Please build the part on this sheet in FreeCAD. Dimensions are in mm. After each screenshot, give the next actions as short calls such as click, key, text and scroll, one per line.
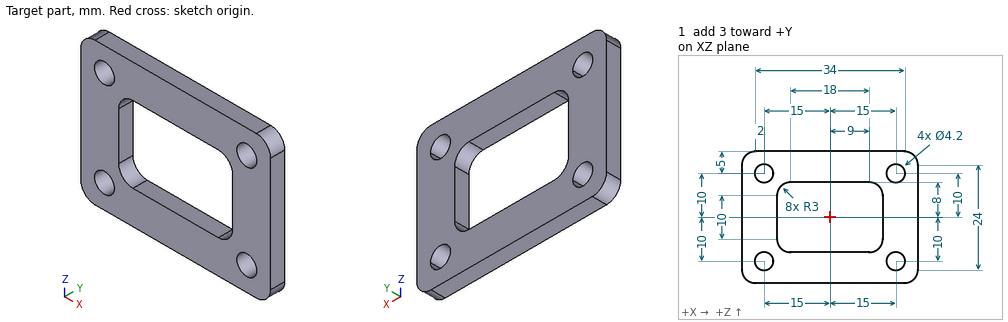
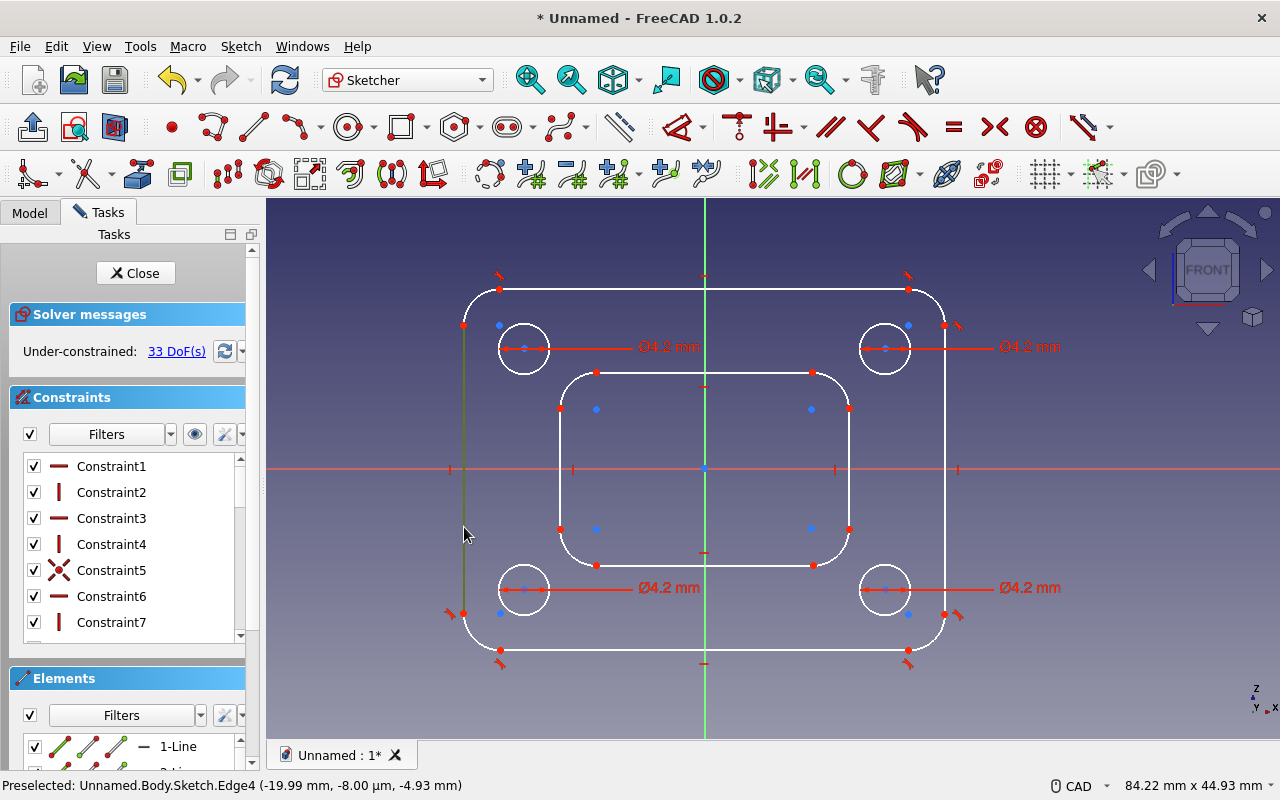
click(484, 293)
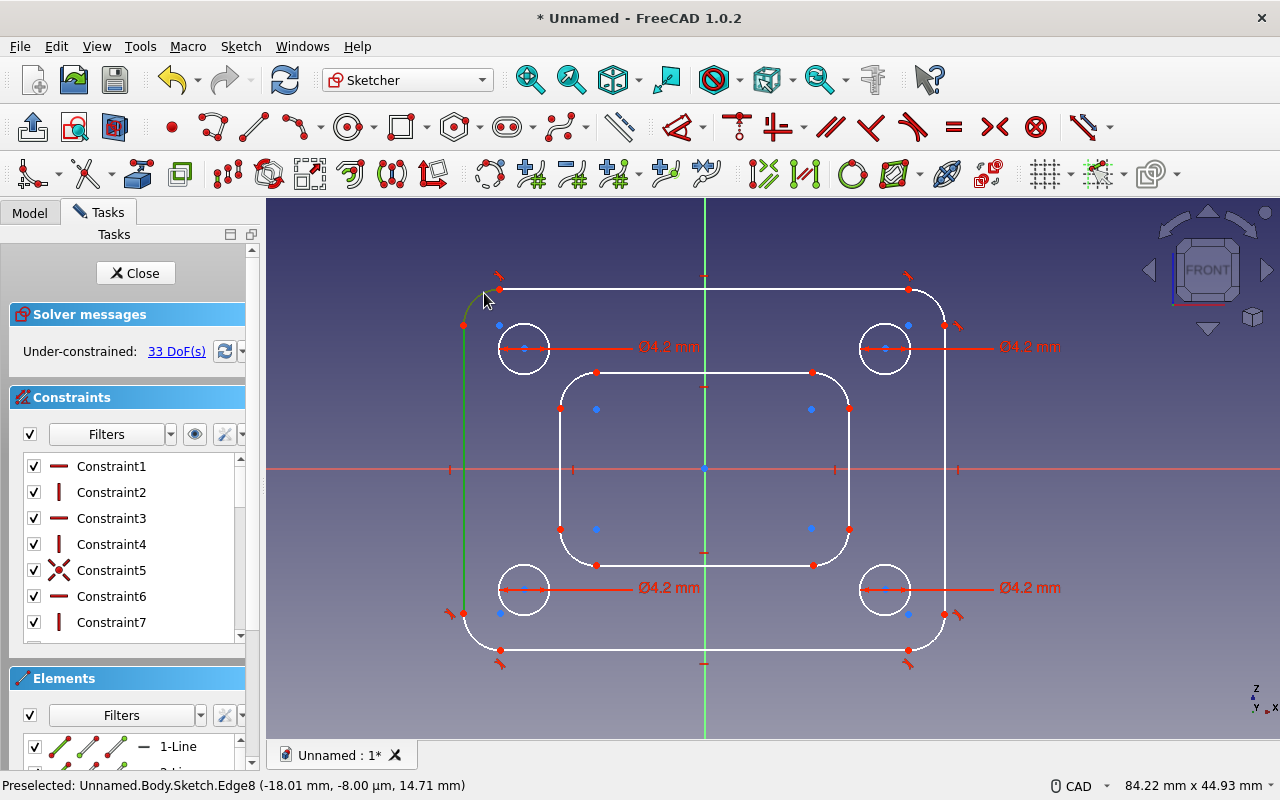
key(t)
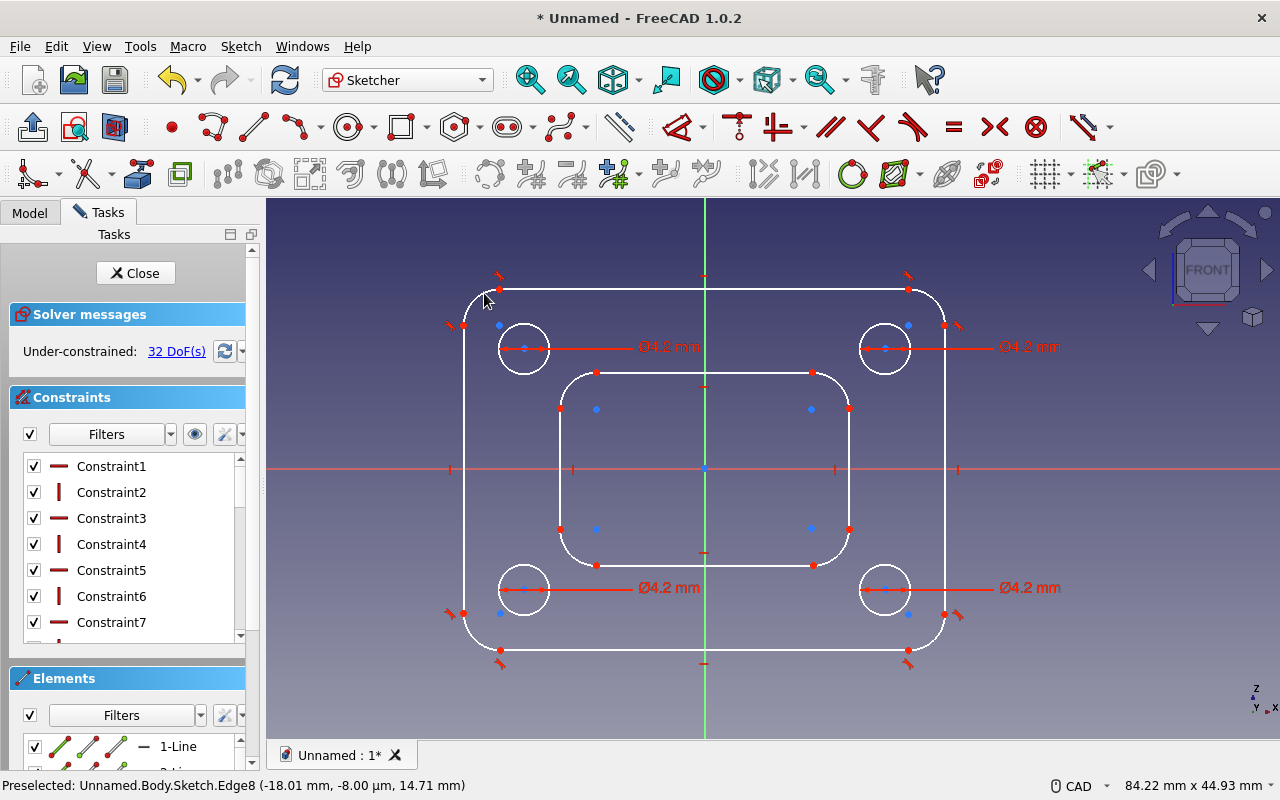
click(748, 373)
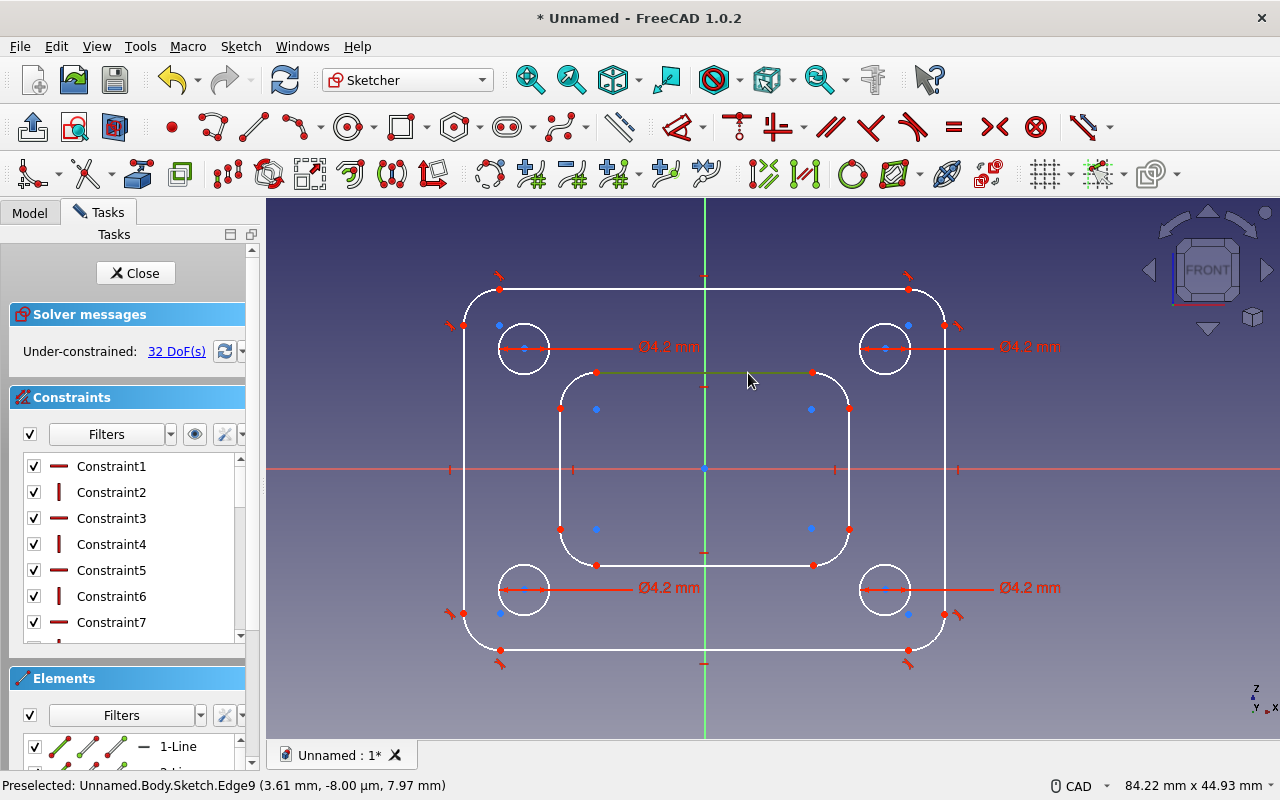
click(580, 377)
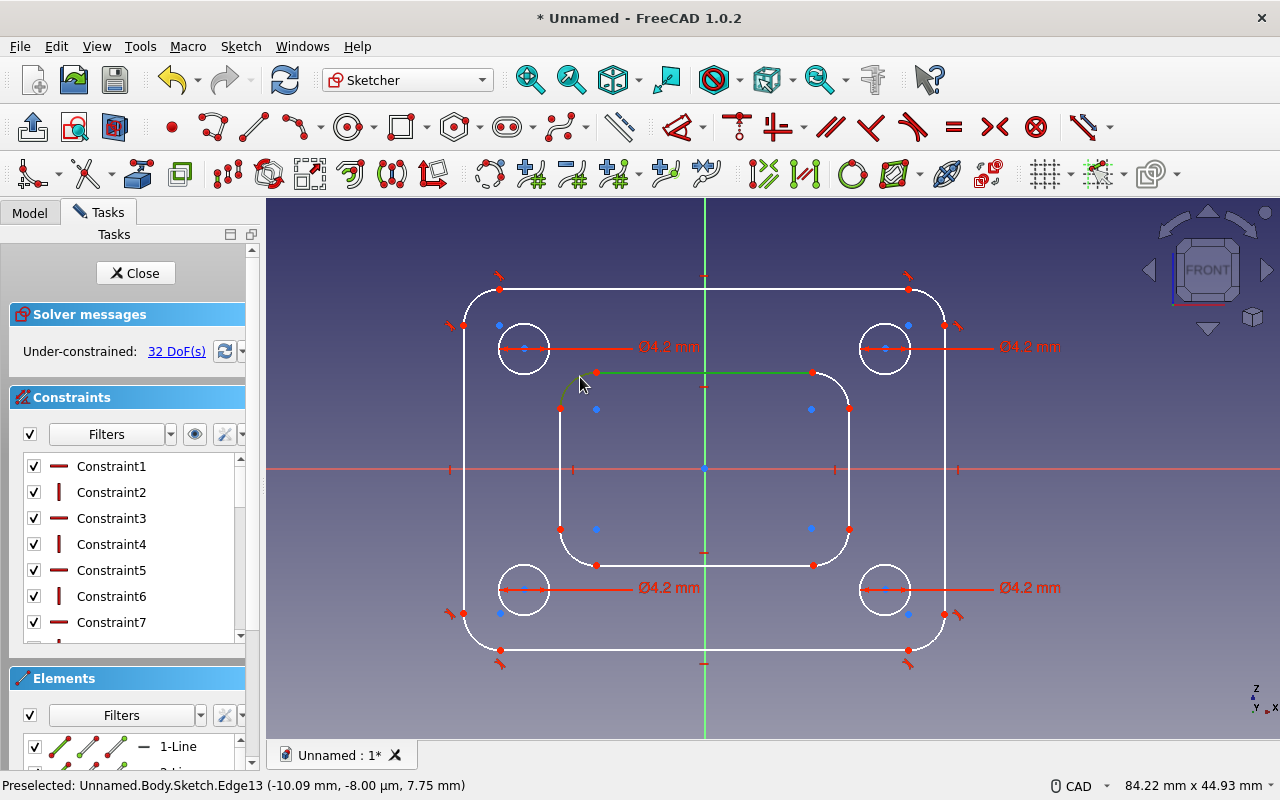
key(t)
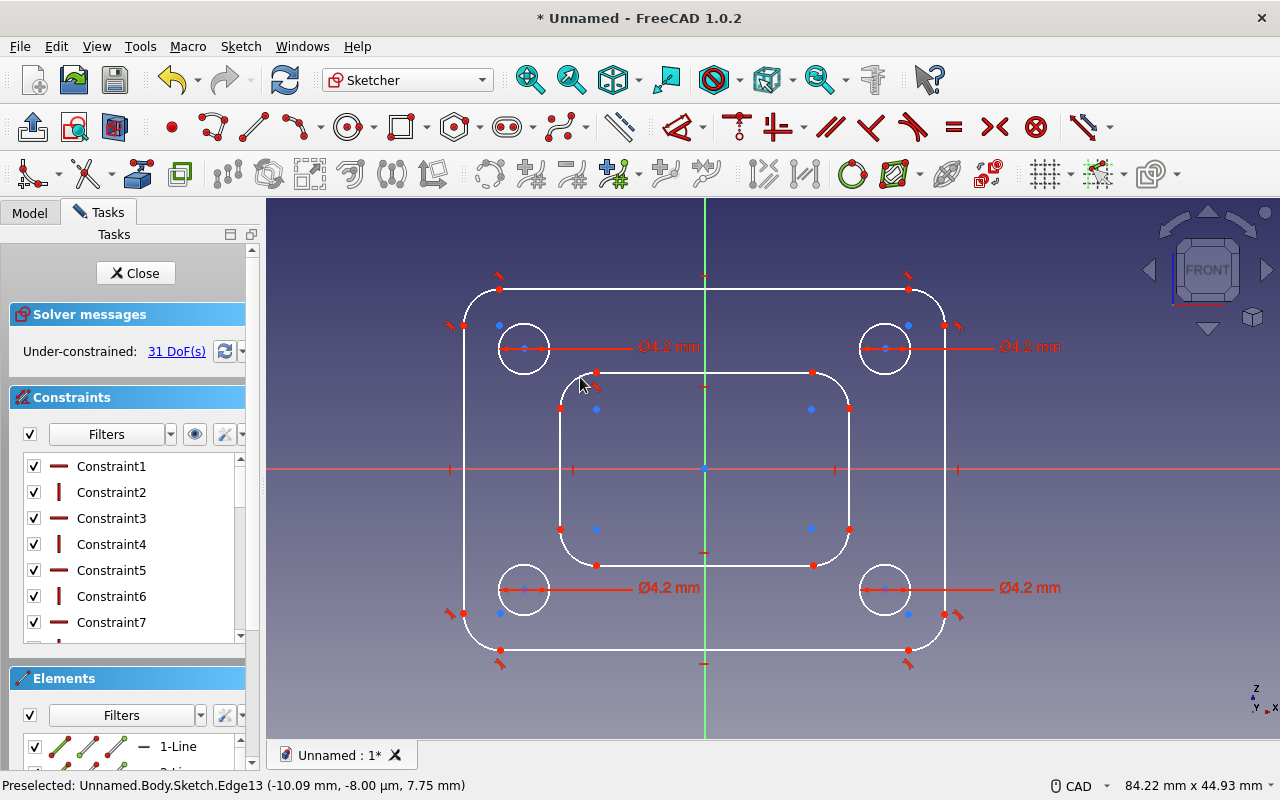
click(748, 373)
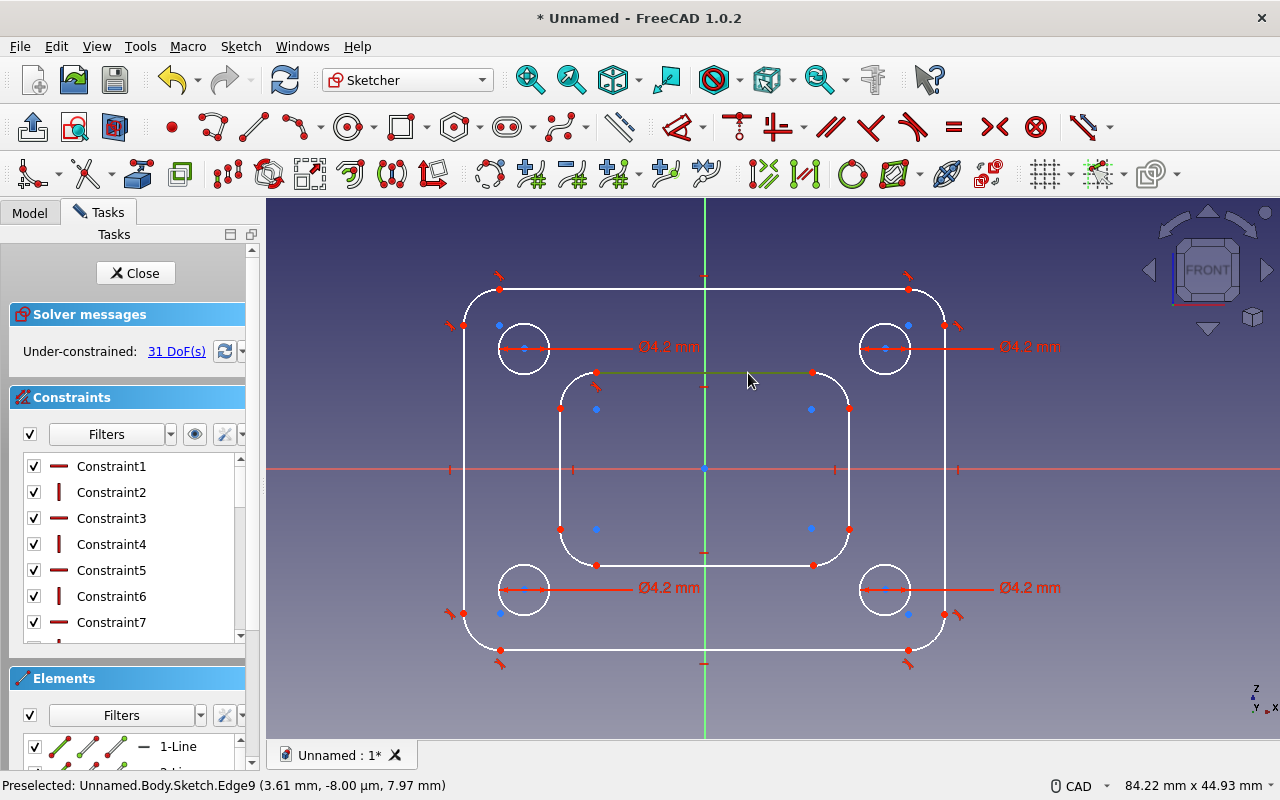
click(845, 393)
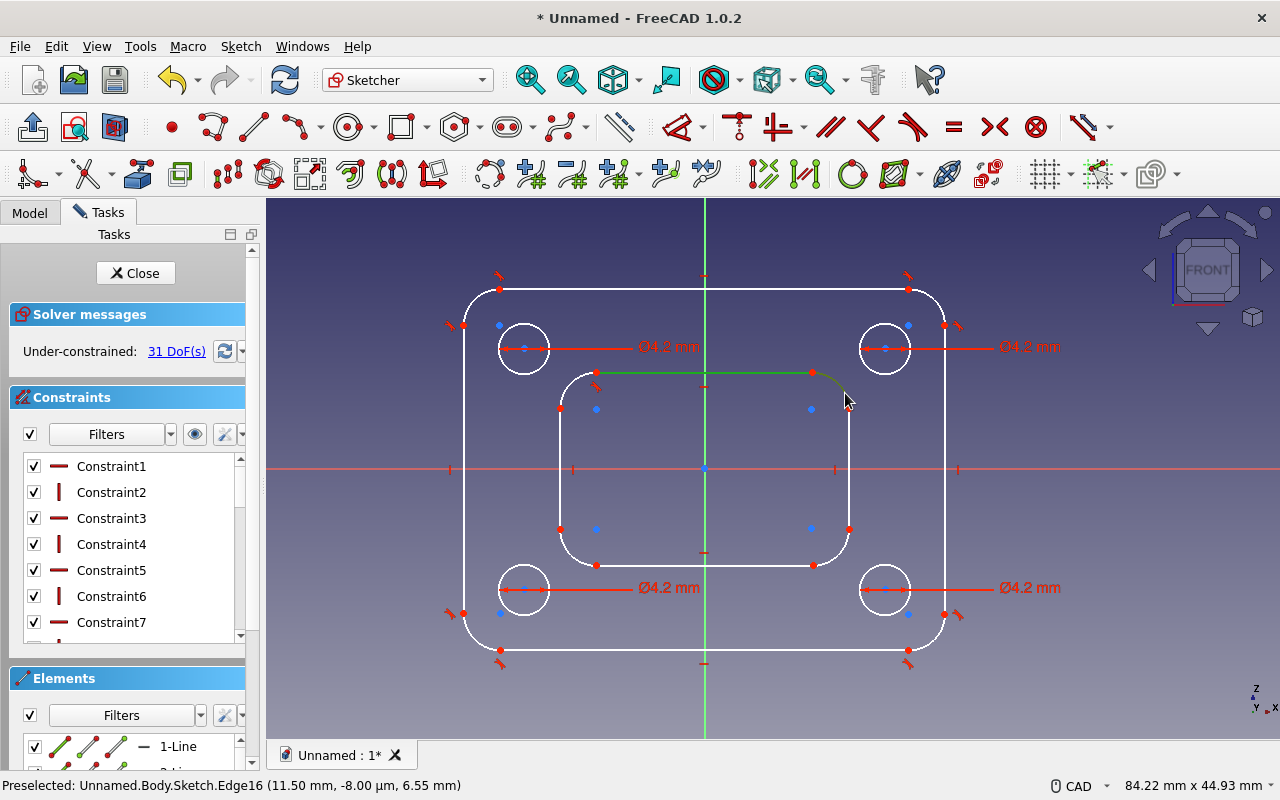
key(t)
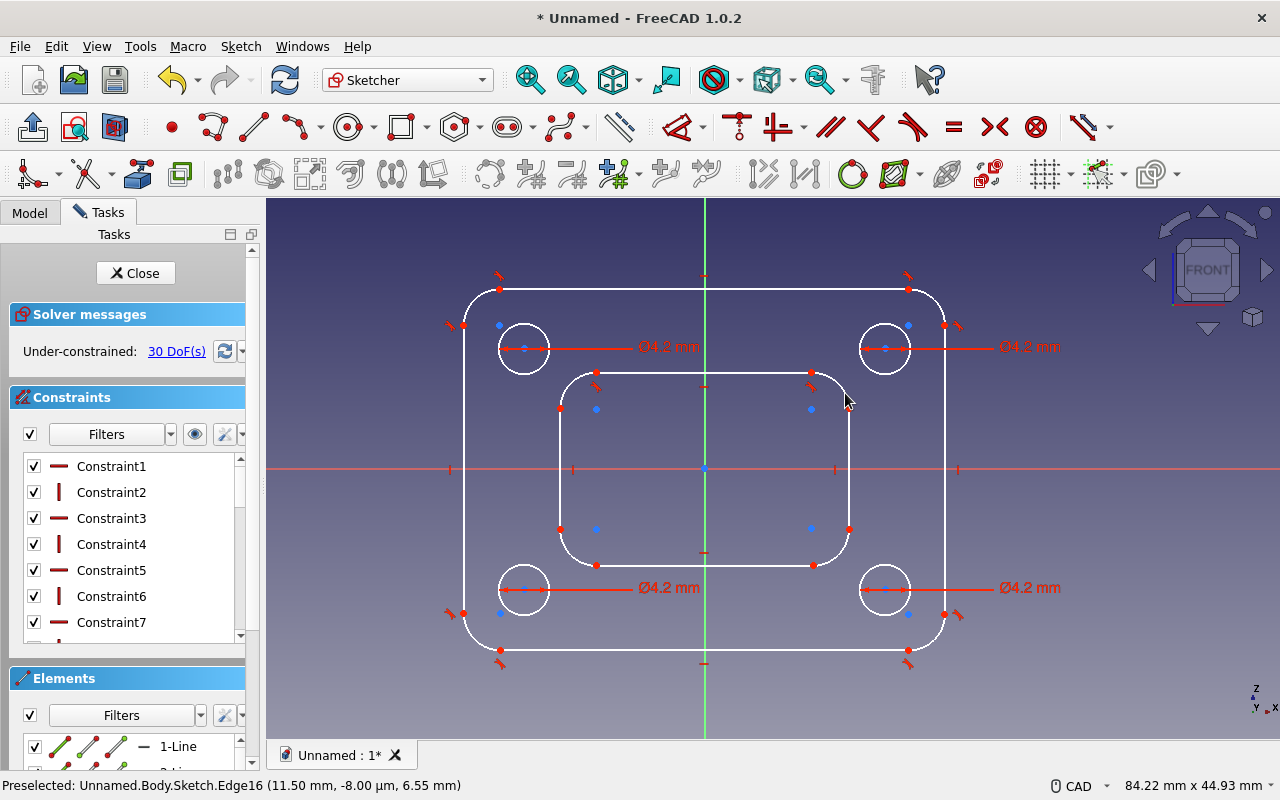
click(560, 445)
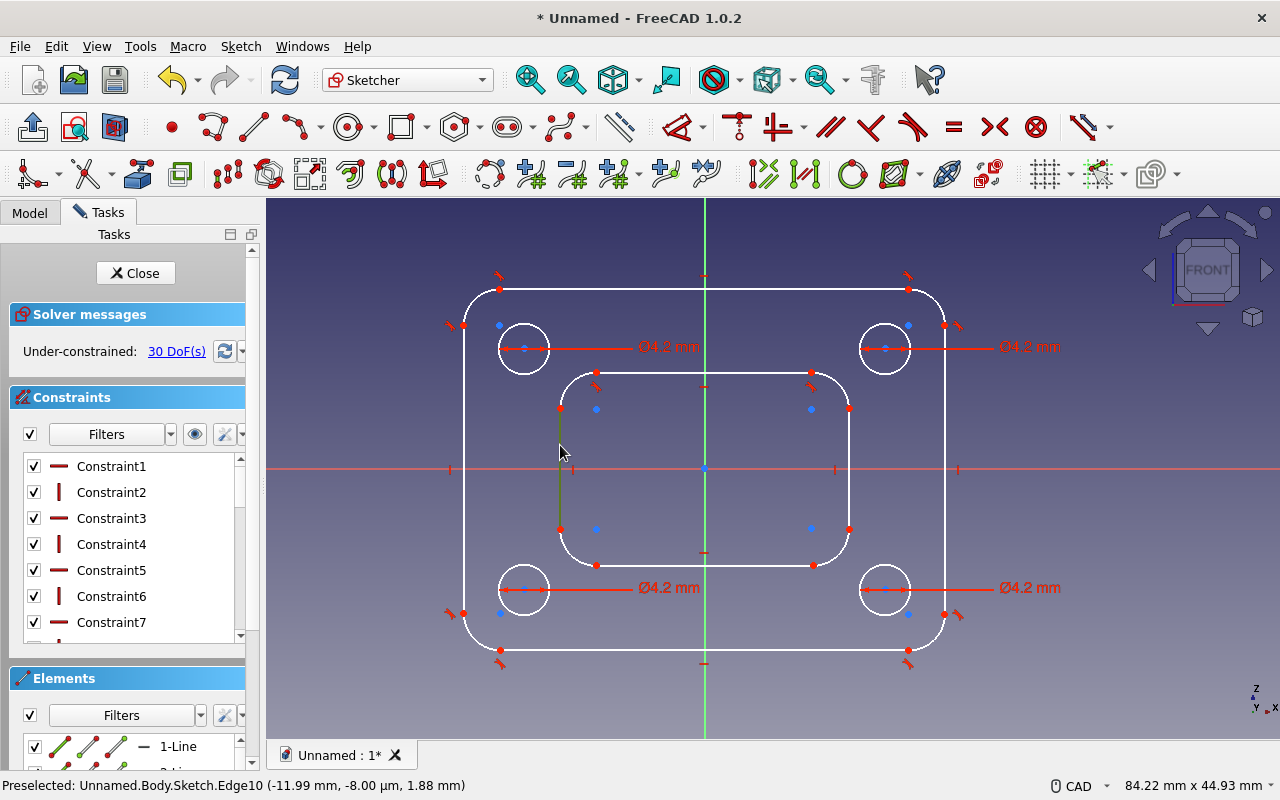
click(580, 377)